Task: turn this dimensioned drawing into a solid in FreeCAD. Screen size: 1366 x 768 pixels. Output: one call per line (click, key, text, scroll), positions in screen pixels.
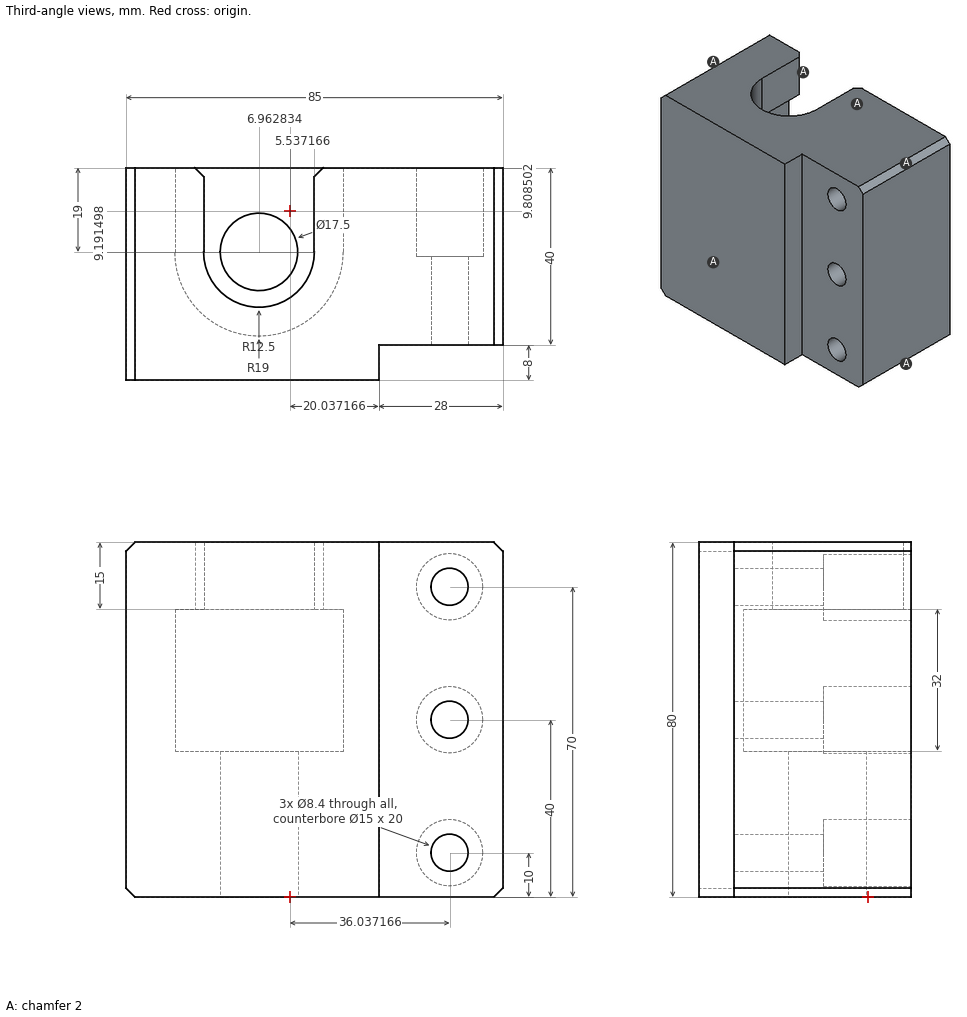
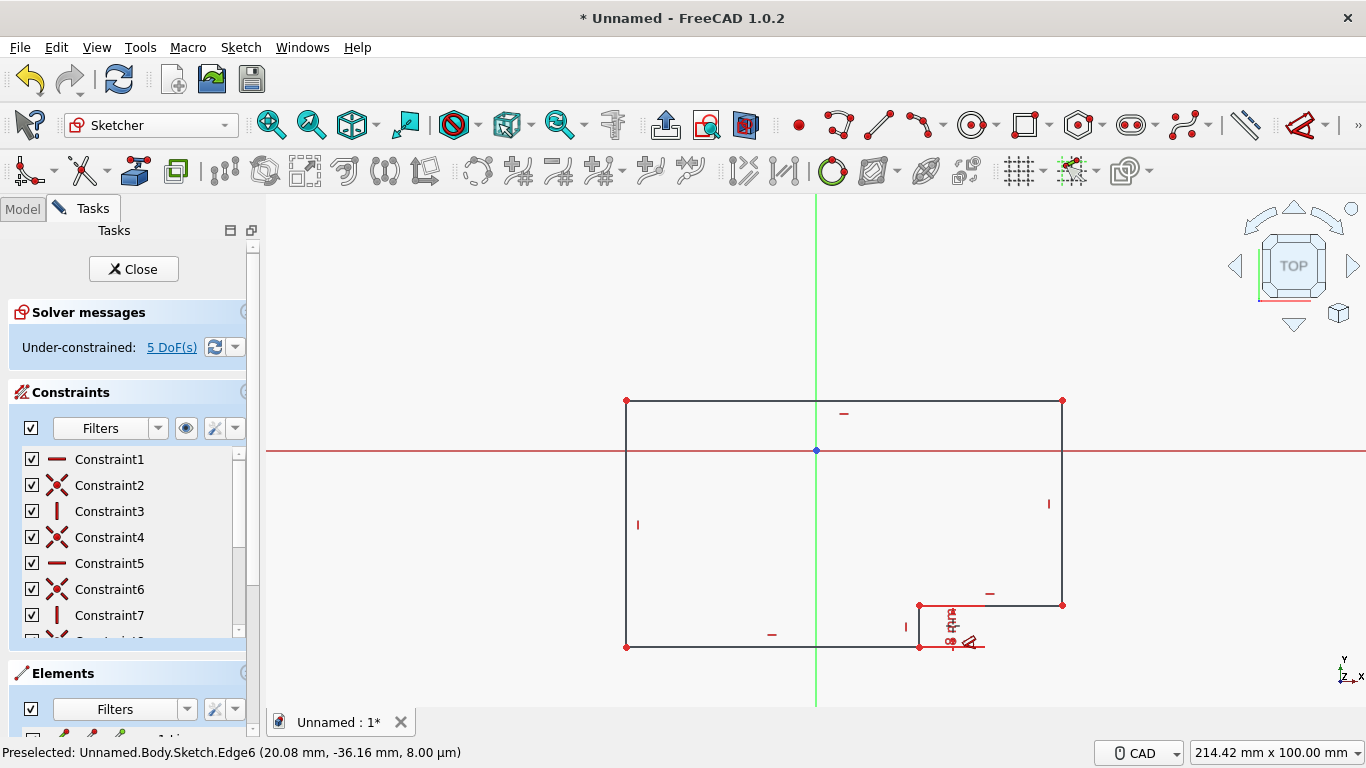
click(962, 606)
click(1023, 640)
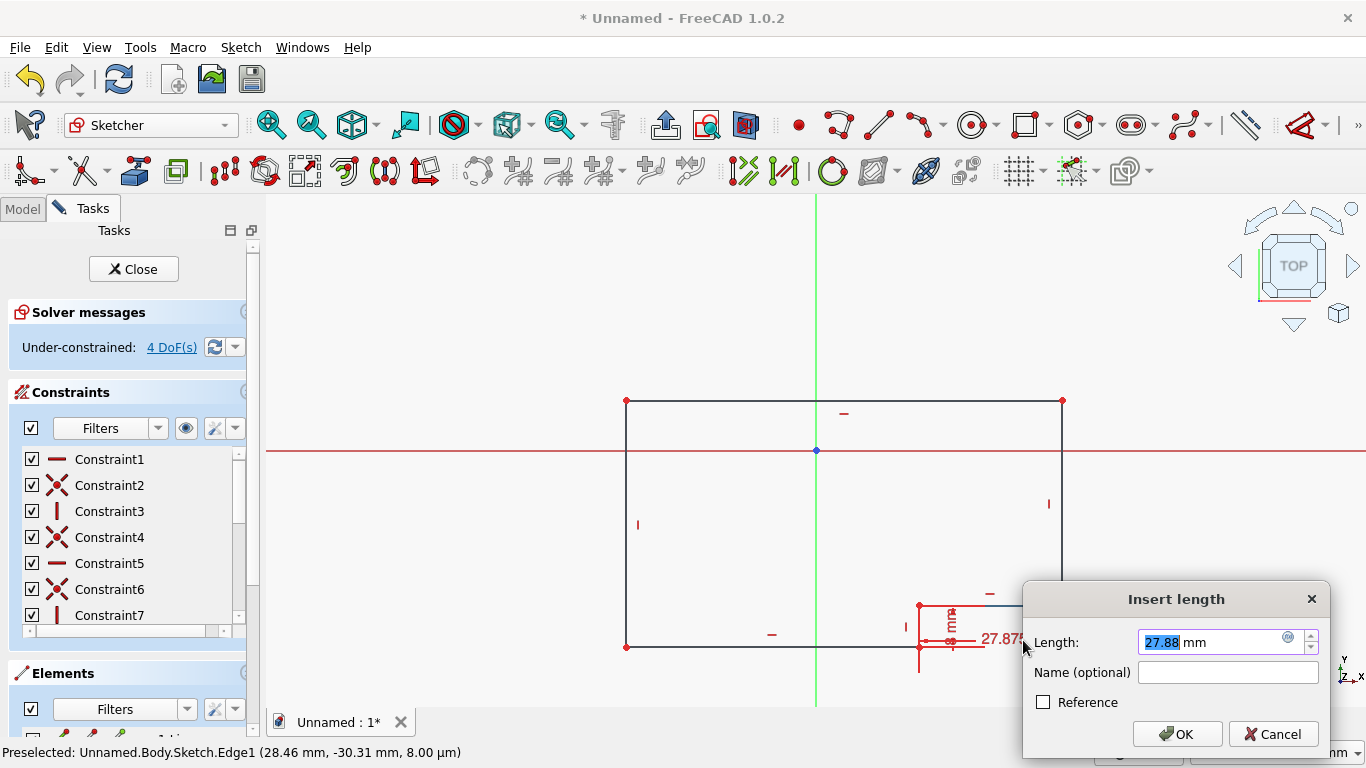
text(28)
key(Return)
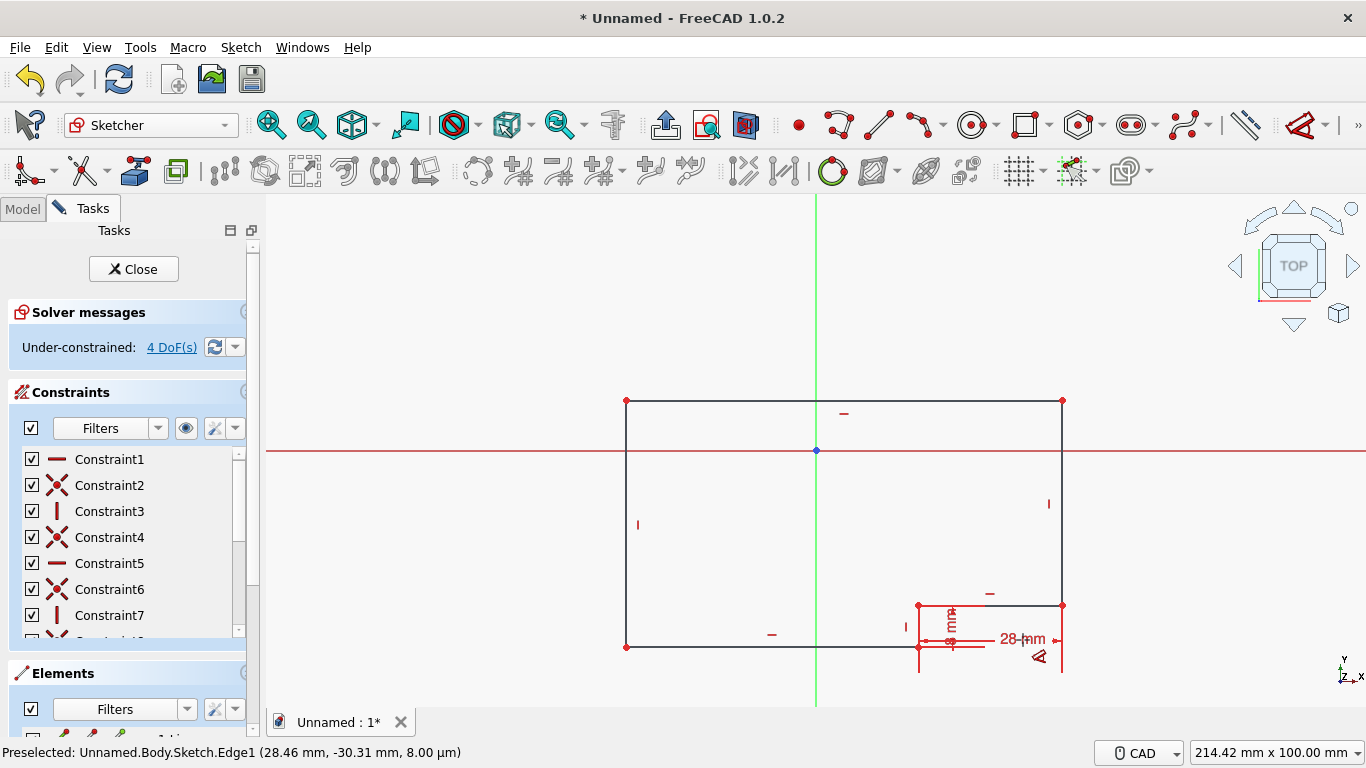
click(1062, 545)
click(1096, 504)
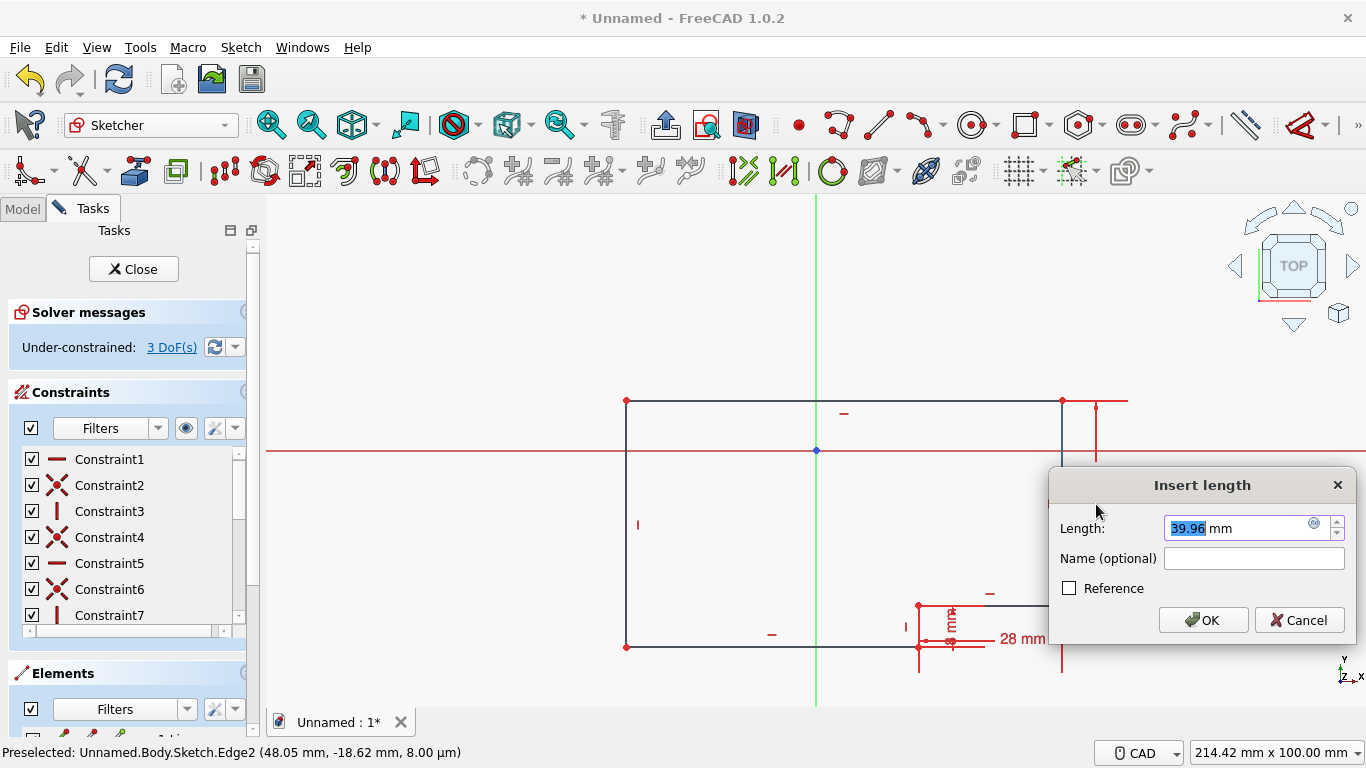
text(40)
key(Return)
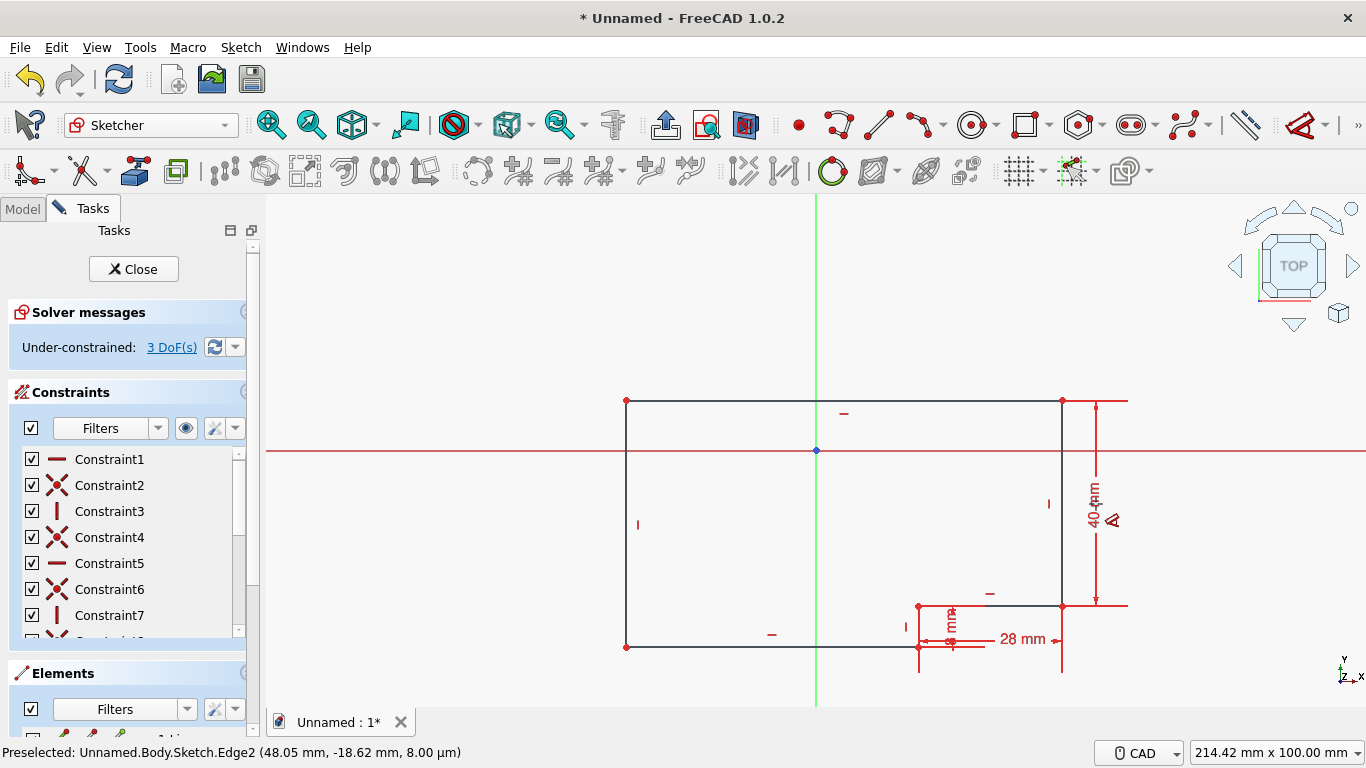
click(932, 401)
click(844, 367)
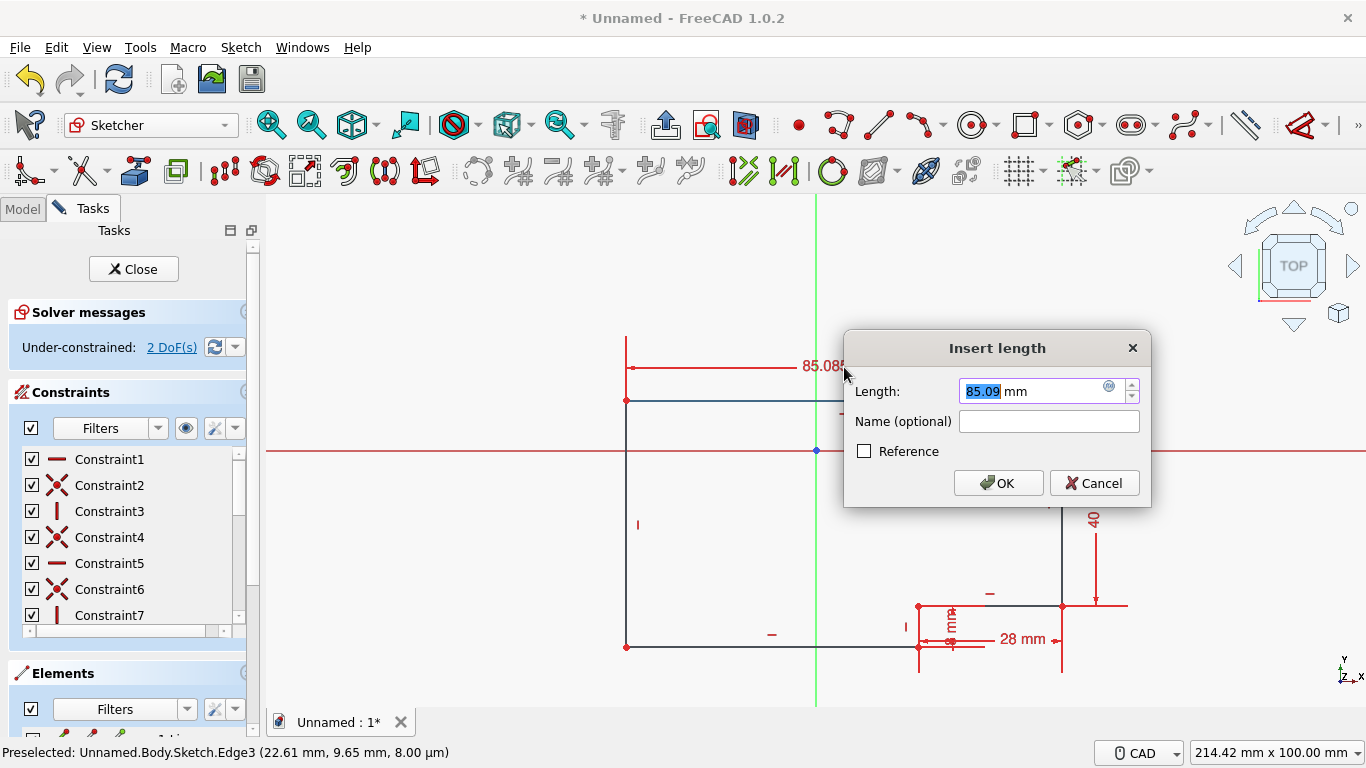
text(85)
key(Return)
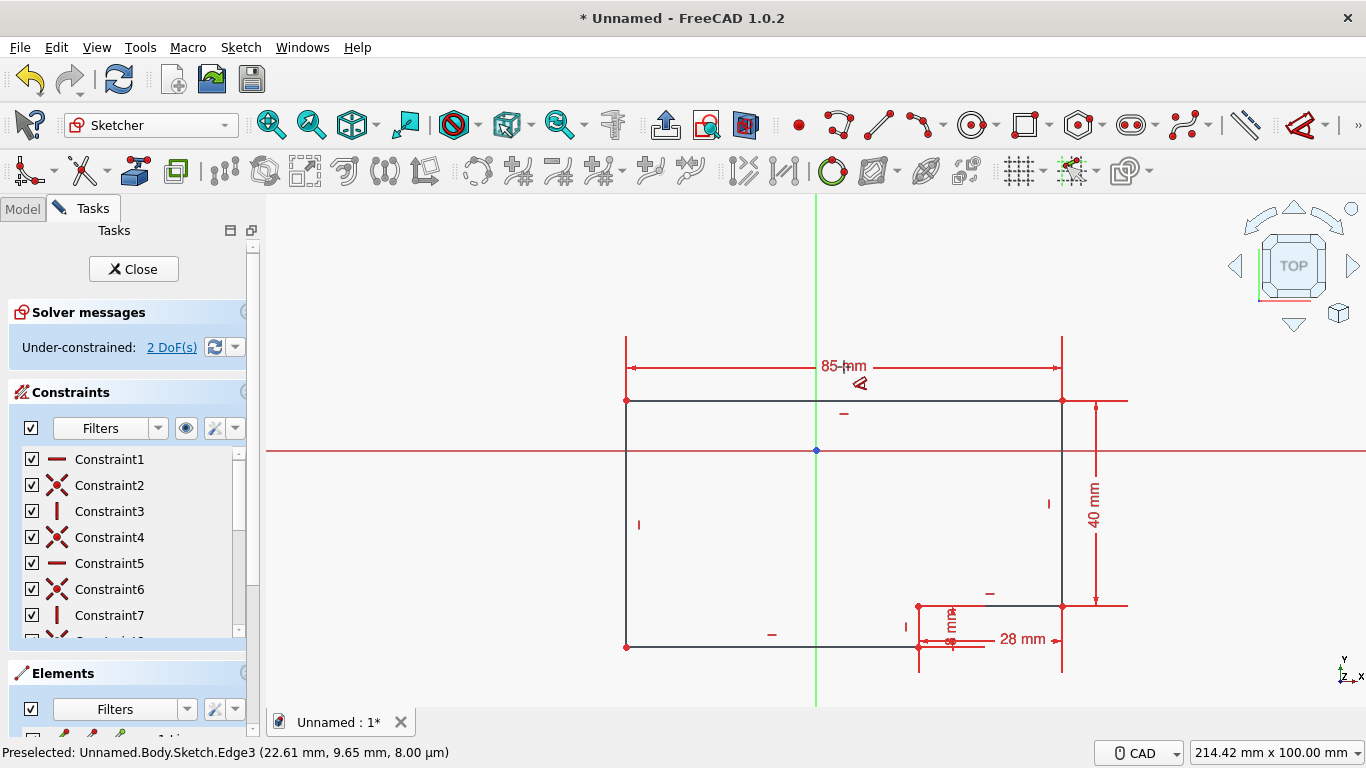
click(1062, 401)
click(1096, 426)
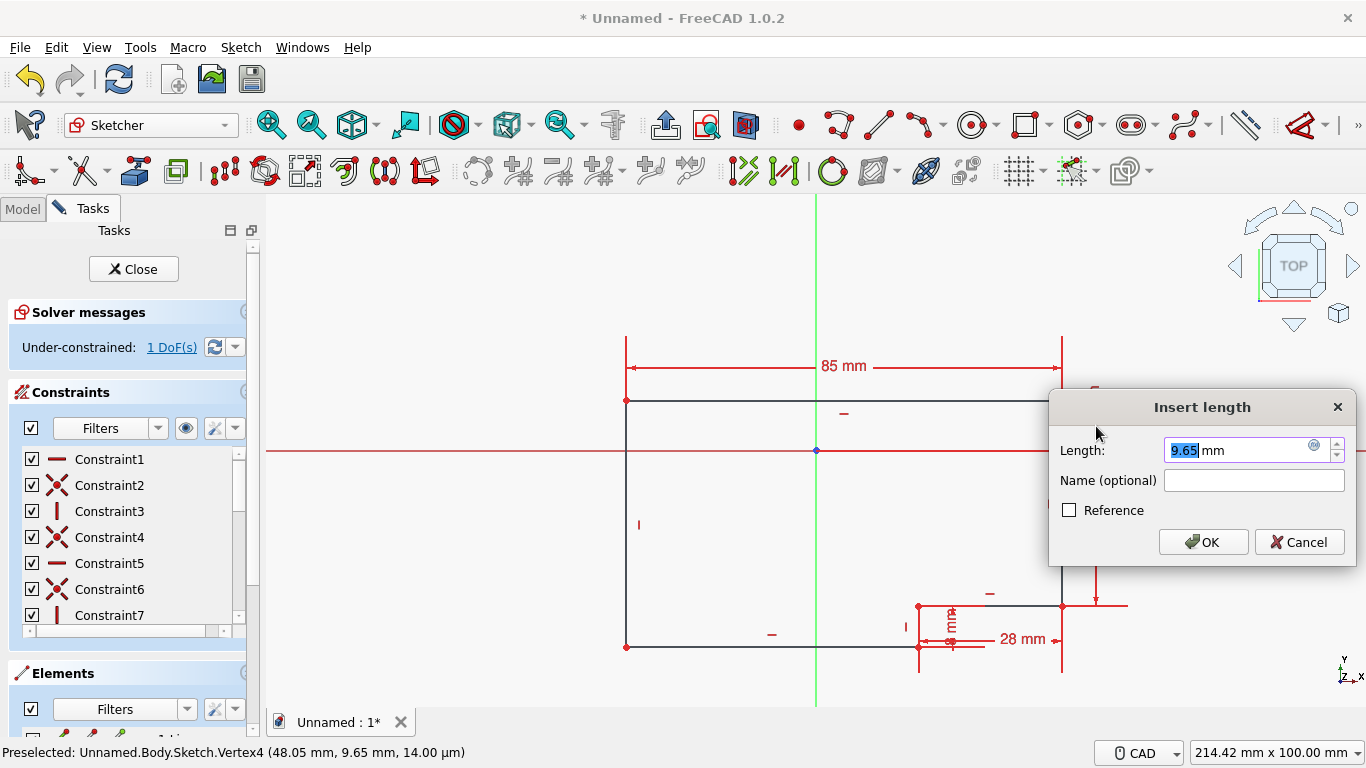
text(9.808502)
key(Return)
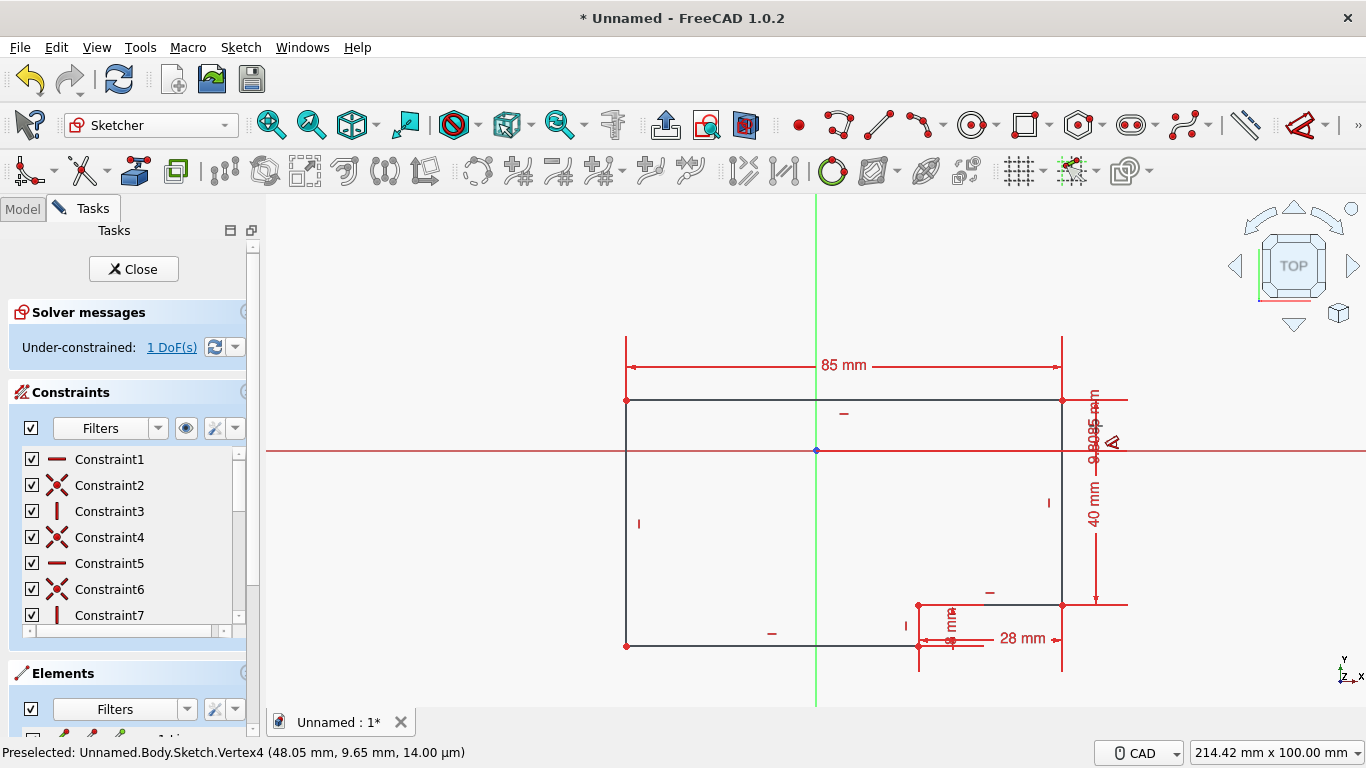
click(919, 605)
click(867, 416)